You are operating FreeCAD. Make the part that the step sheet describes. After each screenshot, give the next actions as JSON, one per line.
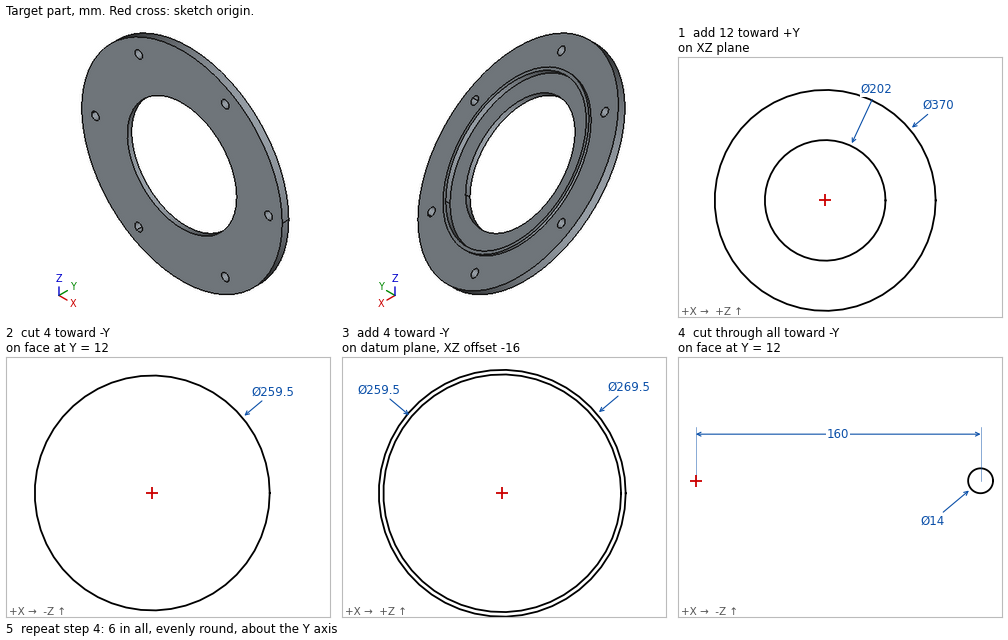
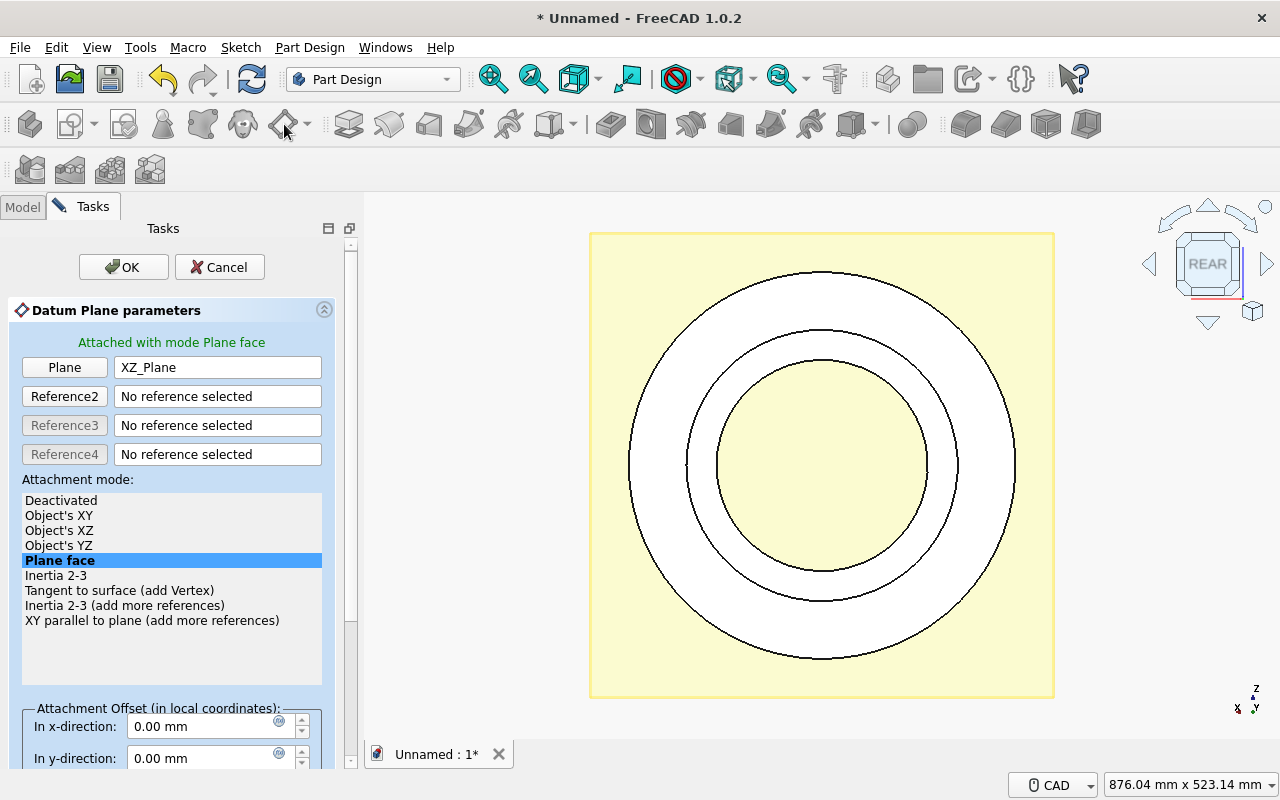
{"action": "scroll", "coordinate": [351, 503], "scroll_direction": "down", "scroll_amount": 2}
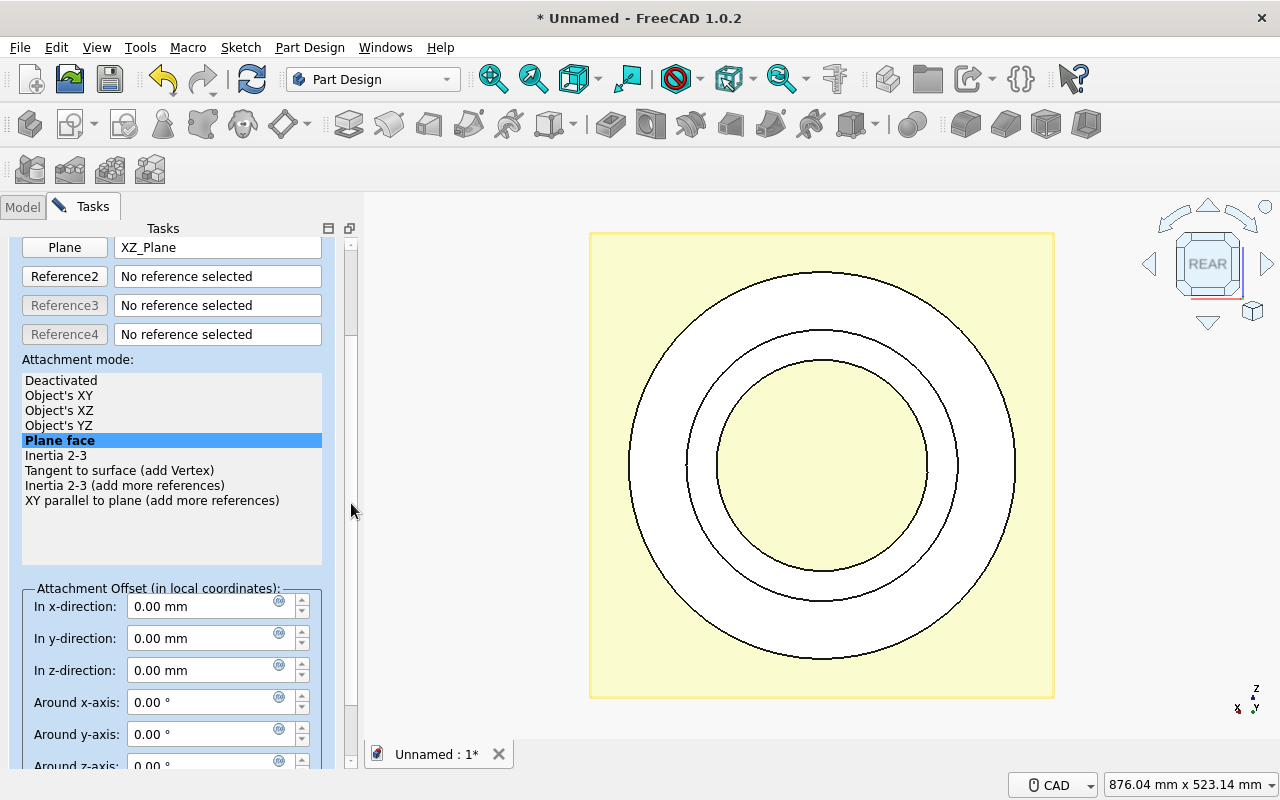
{"action": "triple_click", "coordinate": [210, 670]}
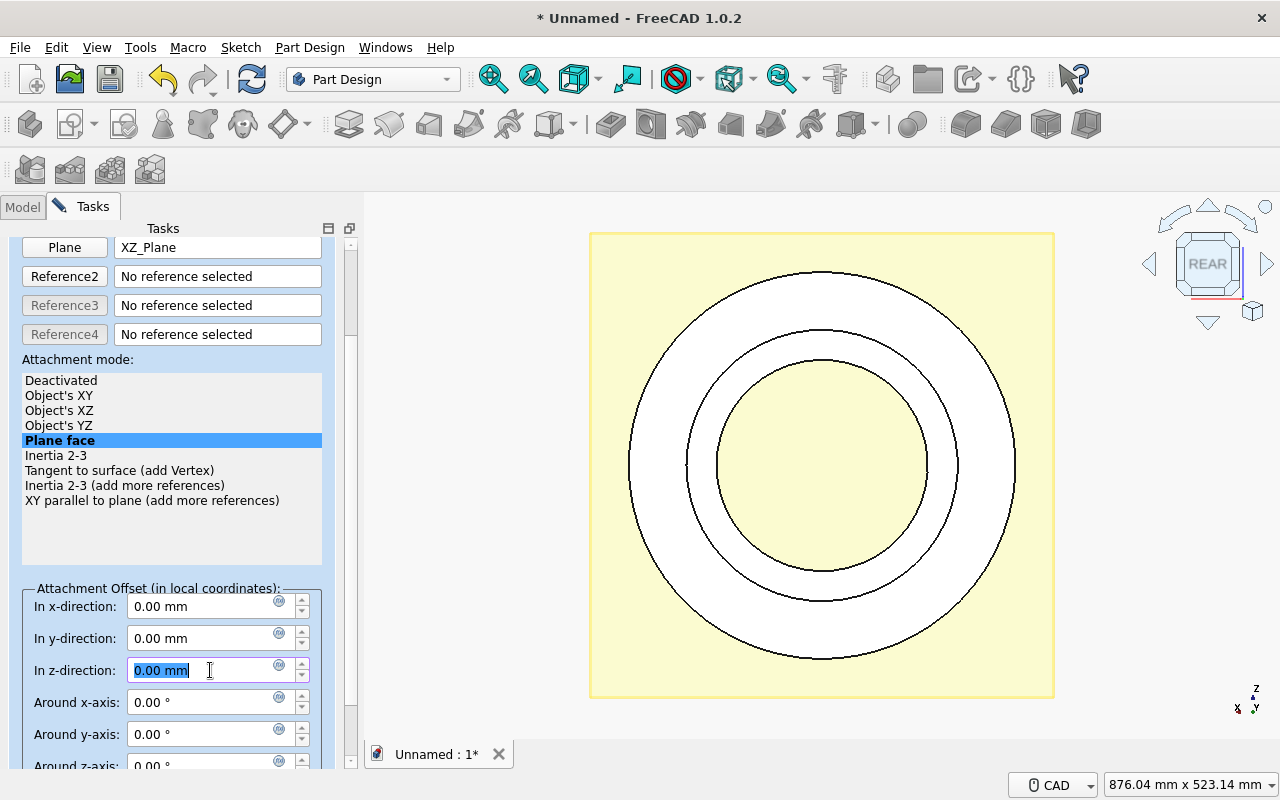
{"action": "type", "text": "-16"}
{"action": "key", "text": "Tab"}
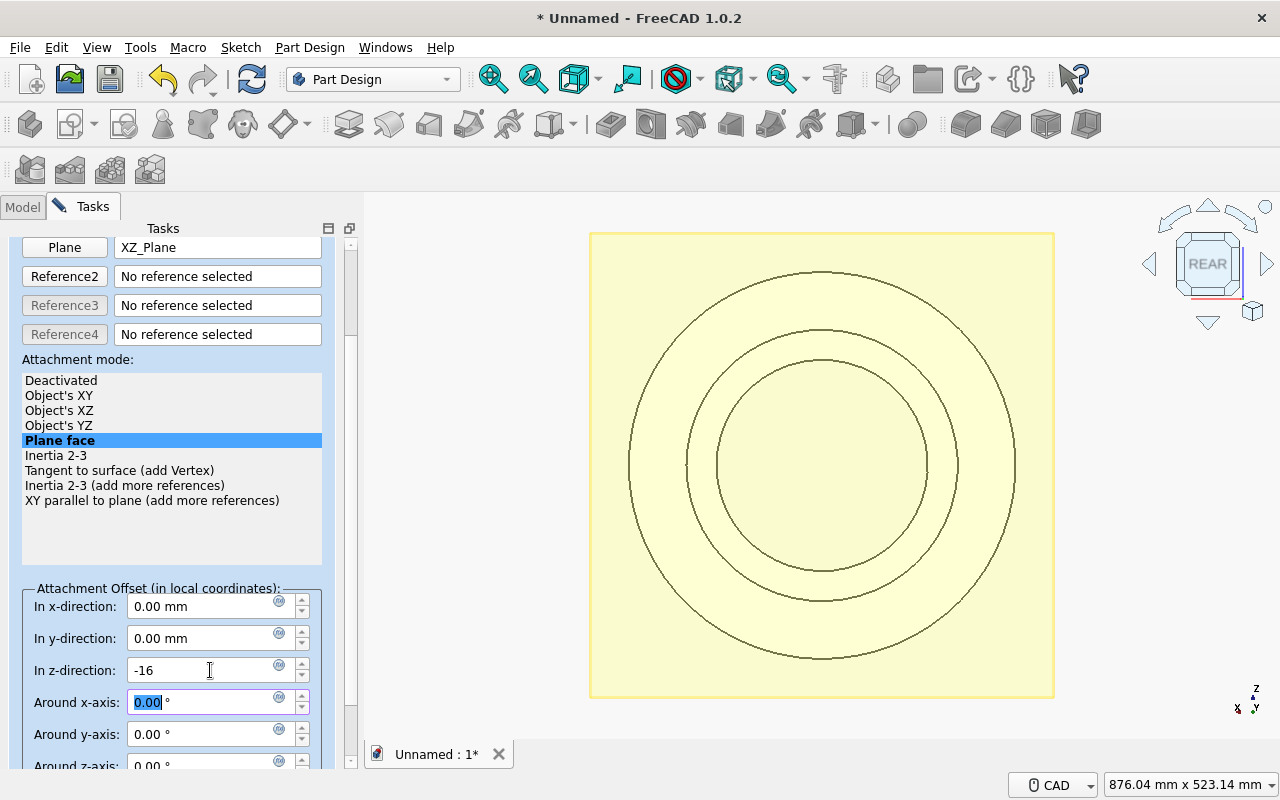
{"action": "scroll", "coordinate": [351, 503], "scroll_direction": "up", "scroll_amount": 3}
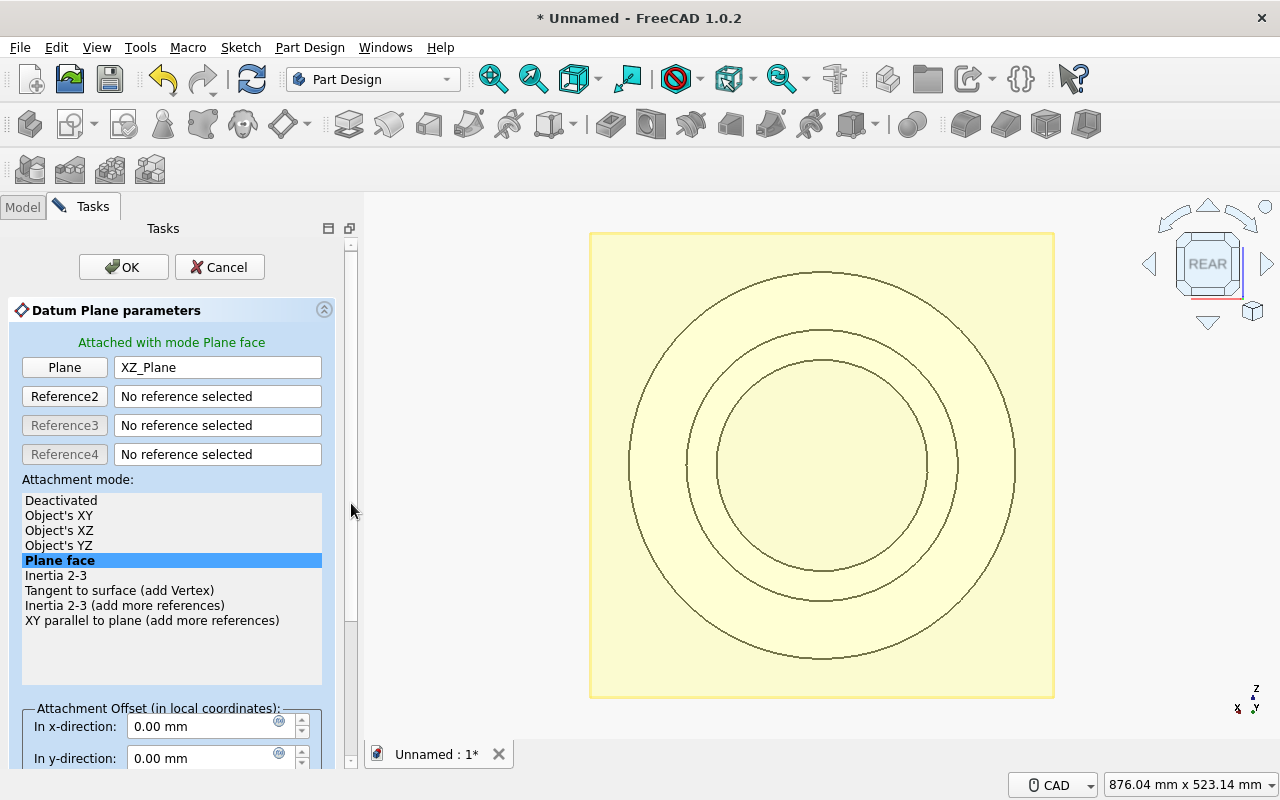
{"action": "left_click", "coordinate": [124, 267]}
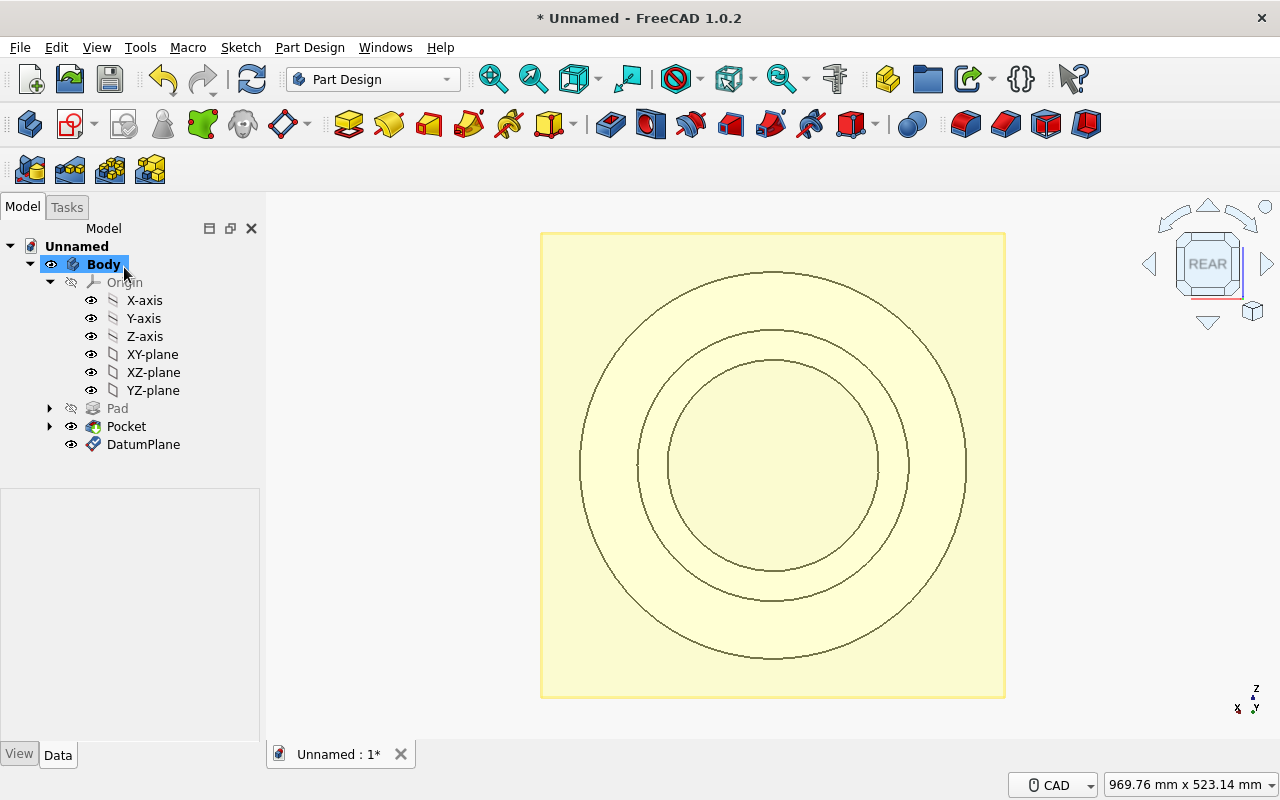
{"action": "left_click", "coordinate": [116, 444]}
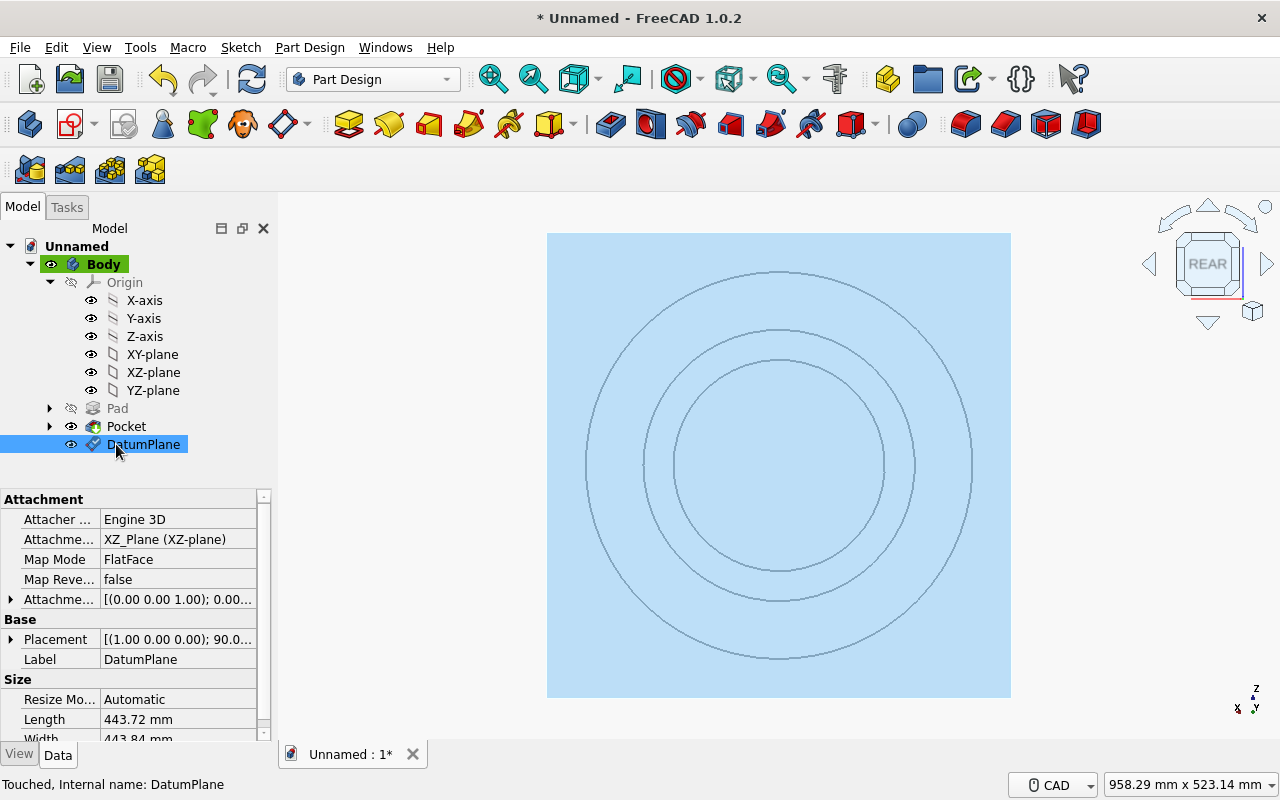
{"action": "left_click", "coordinate": [70, 124]}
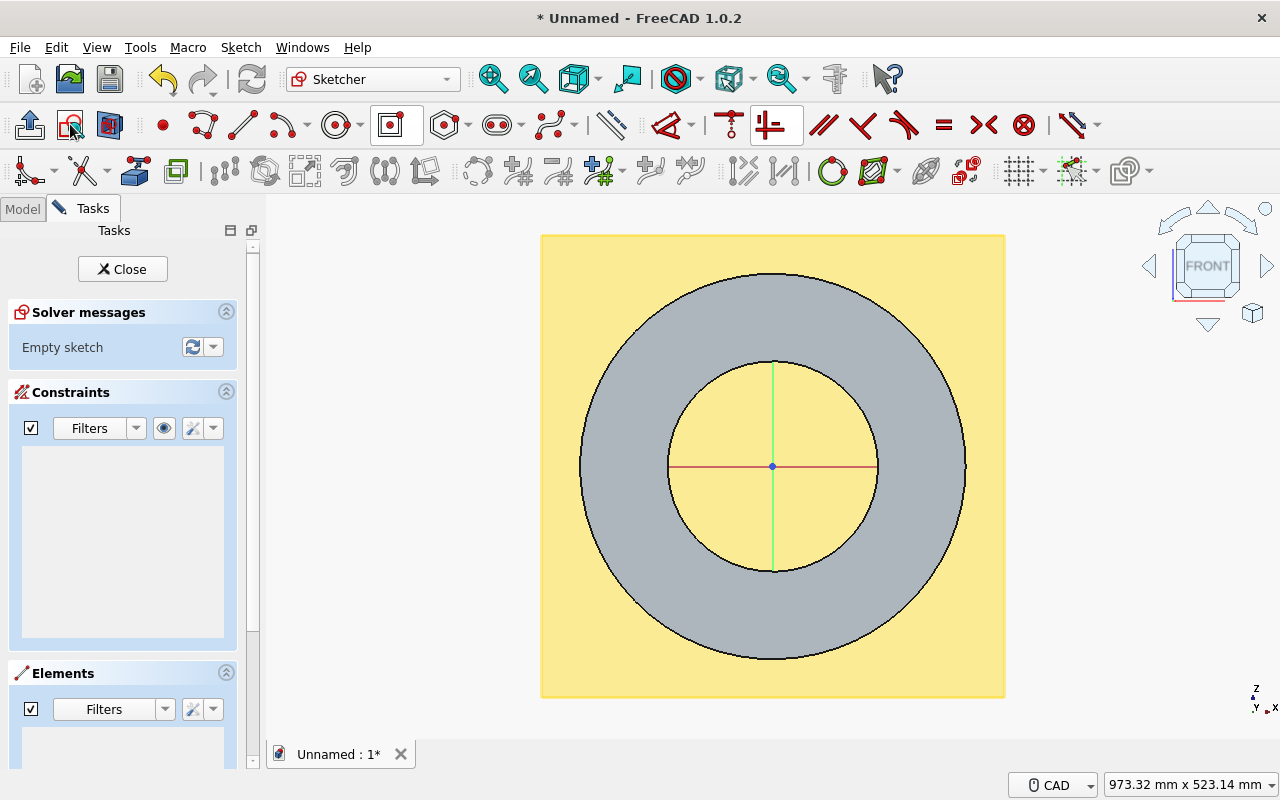
{"action": "left_click", "coordinate": [110, 126]}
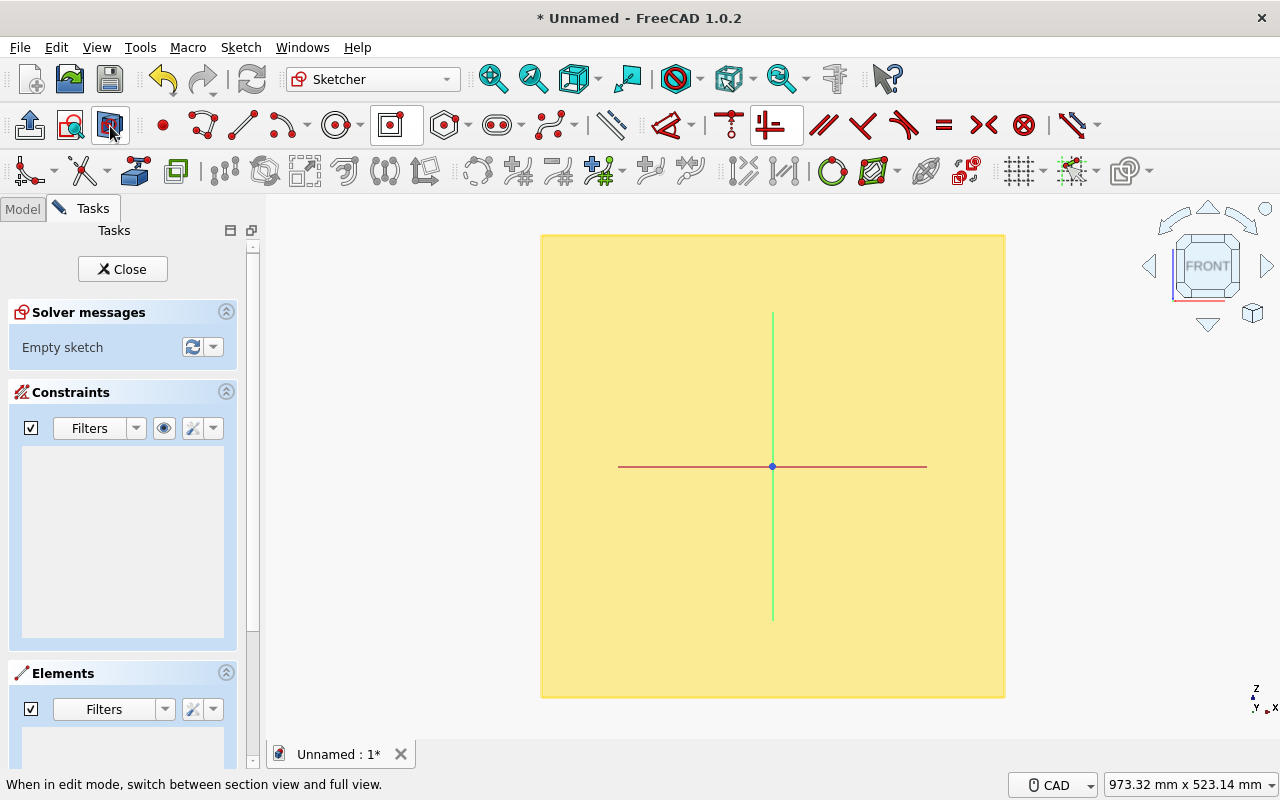
{"action": "left_click", "coordinate": [336, 126]}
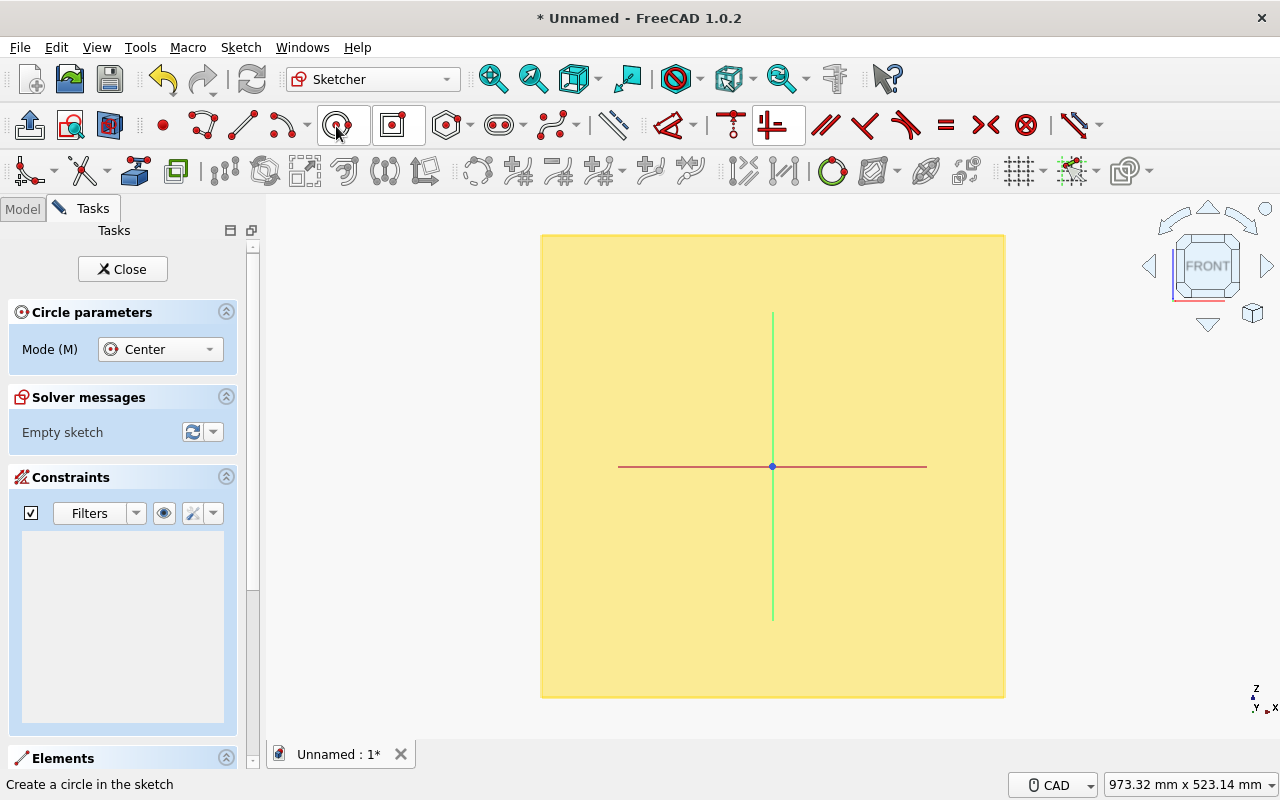
{"action": "left_click", "coordinate": [773, 467]}
{"action": "mouse_move", "coordinate": [872, 367]}